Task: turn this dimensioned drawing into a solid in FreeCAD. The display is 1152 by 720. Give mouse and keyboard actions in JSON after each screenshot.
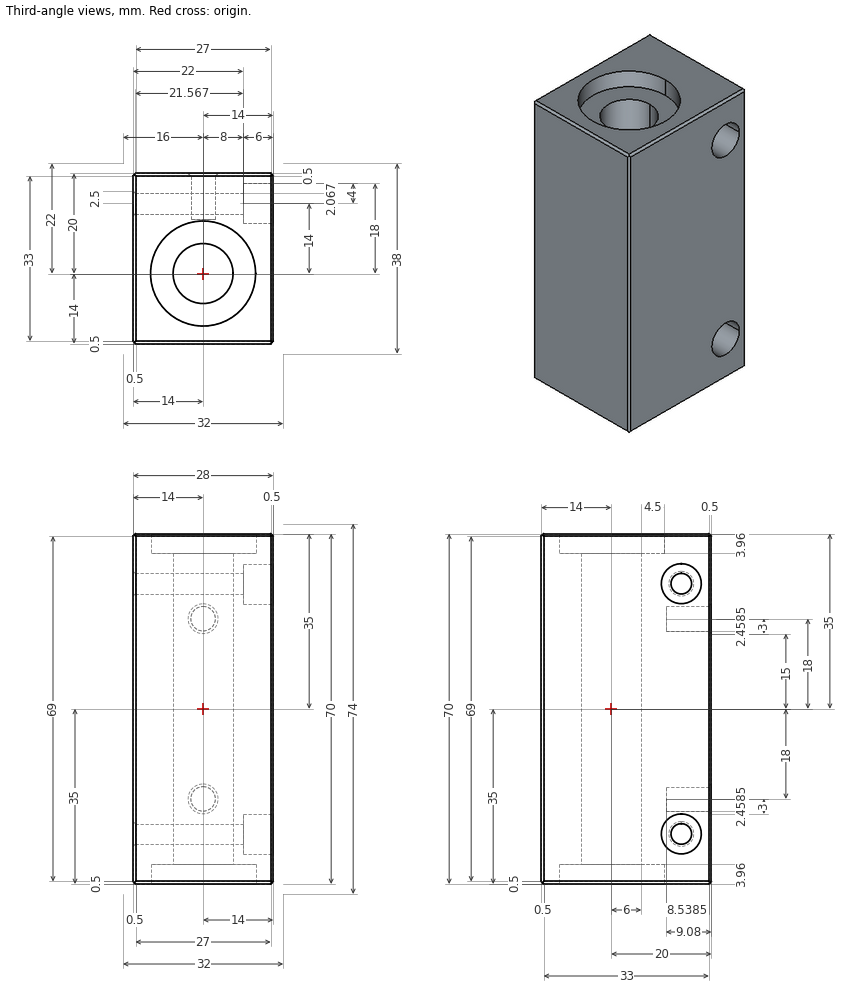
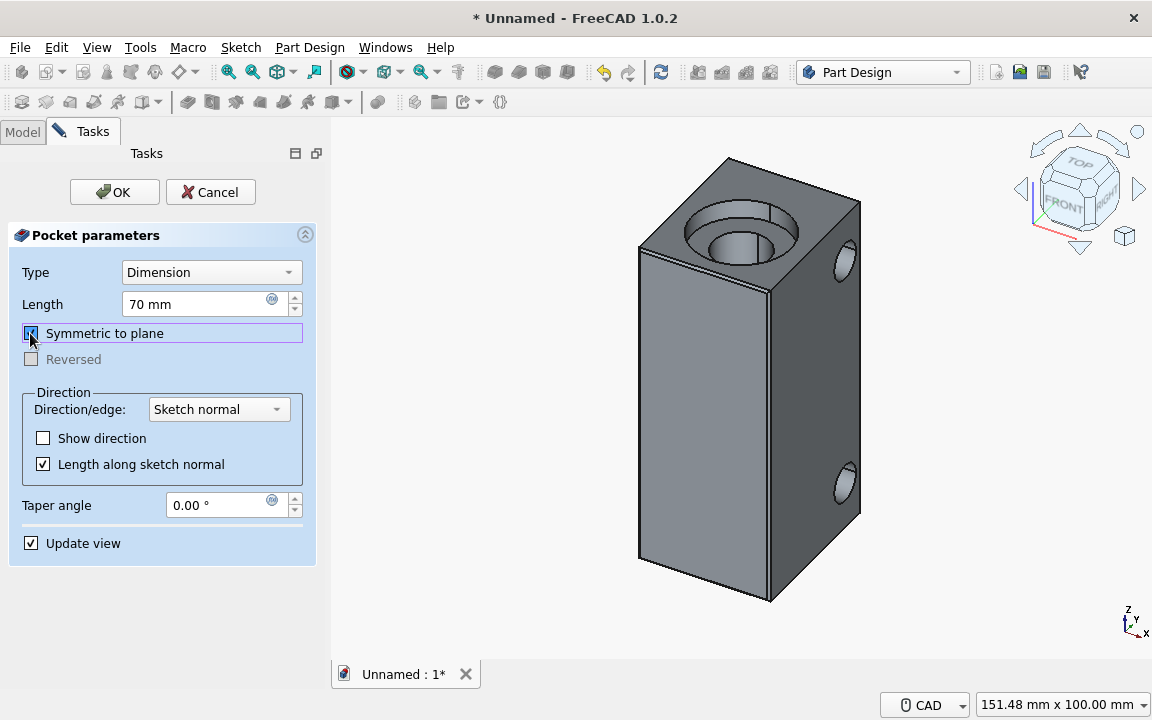
{"action": "left_click", "coordinate": [115, 192]}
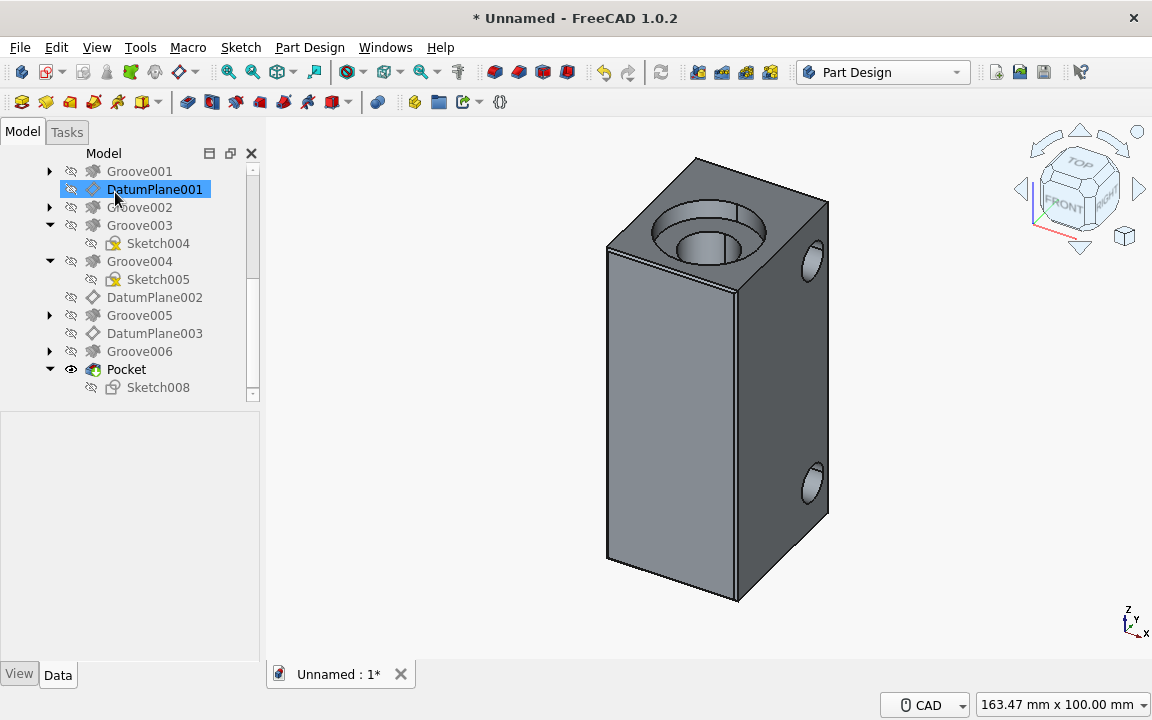
{"action": "left_click", "coordinate": [46, 72]}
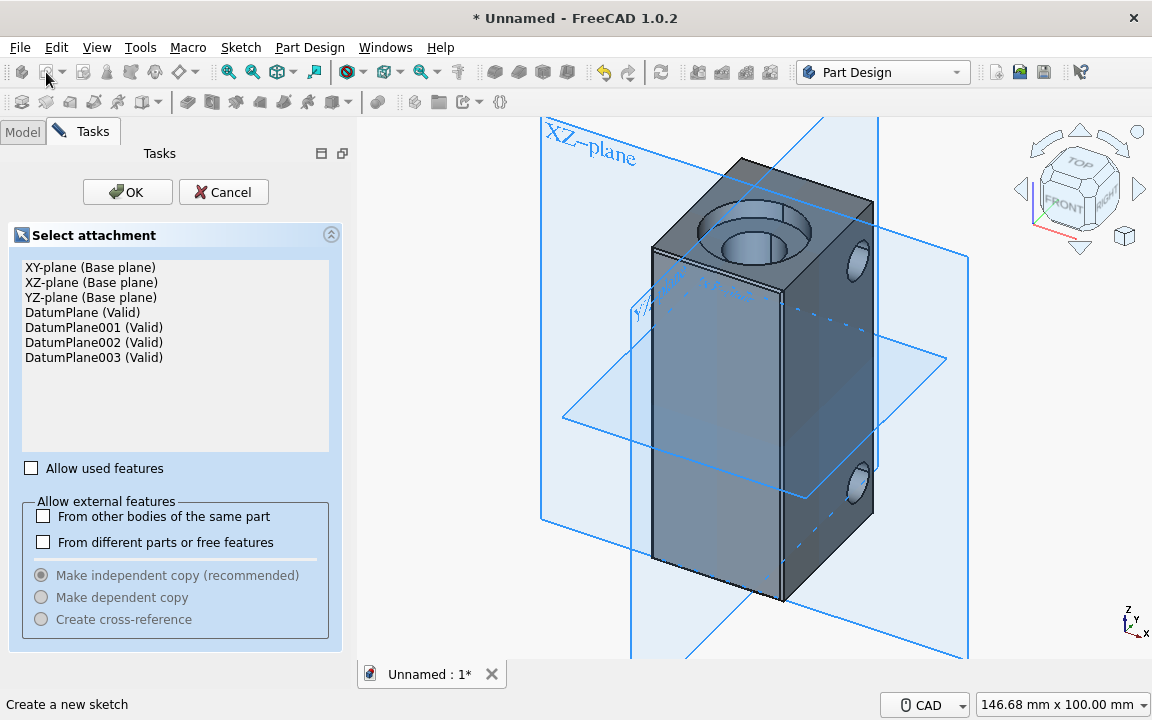
{"action": "left_click", "coordinate": [82, 282]}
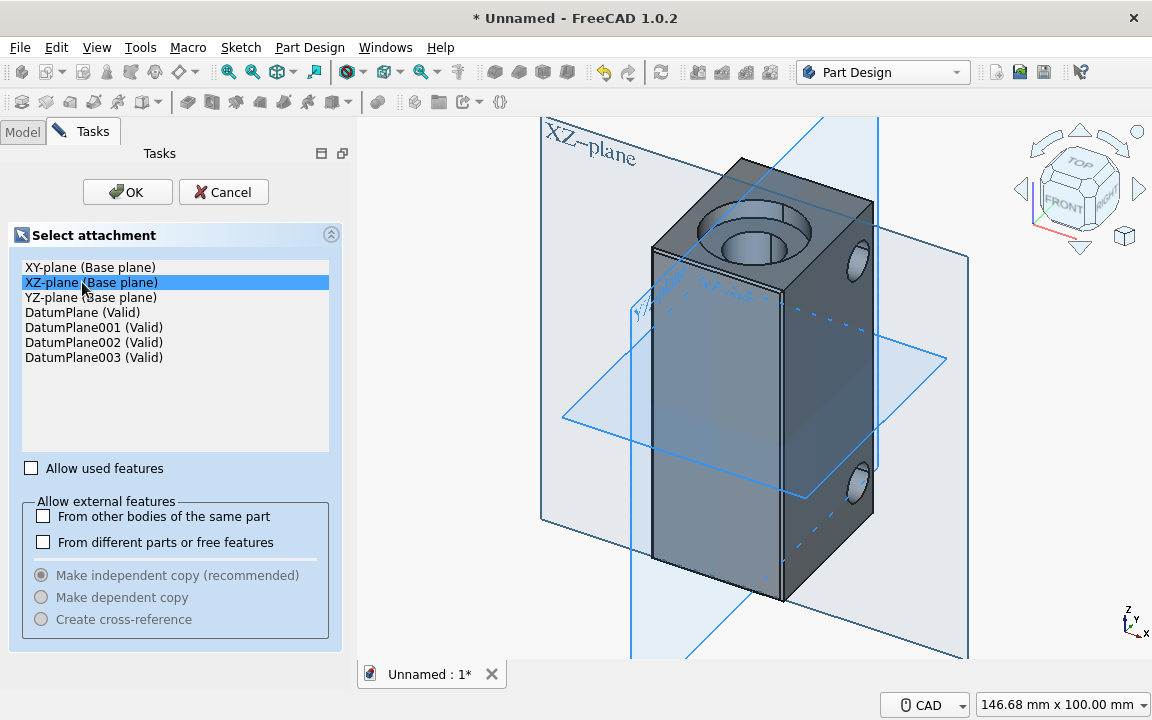
{"action": "left_click", "coordinate": [128, 192]}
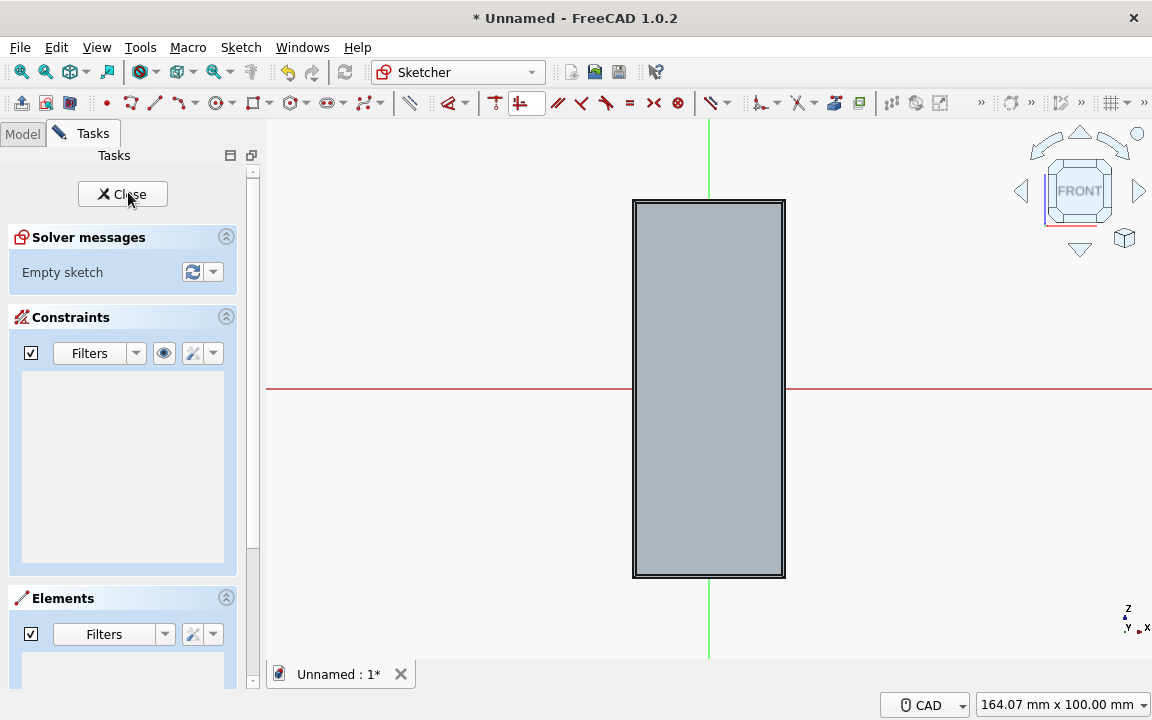
{"action": "left_click", "coordinate": [70, 104]}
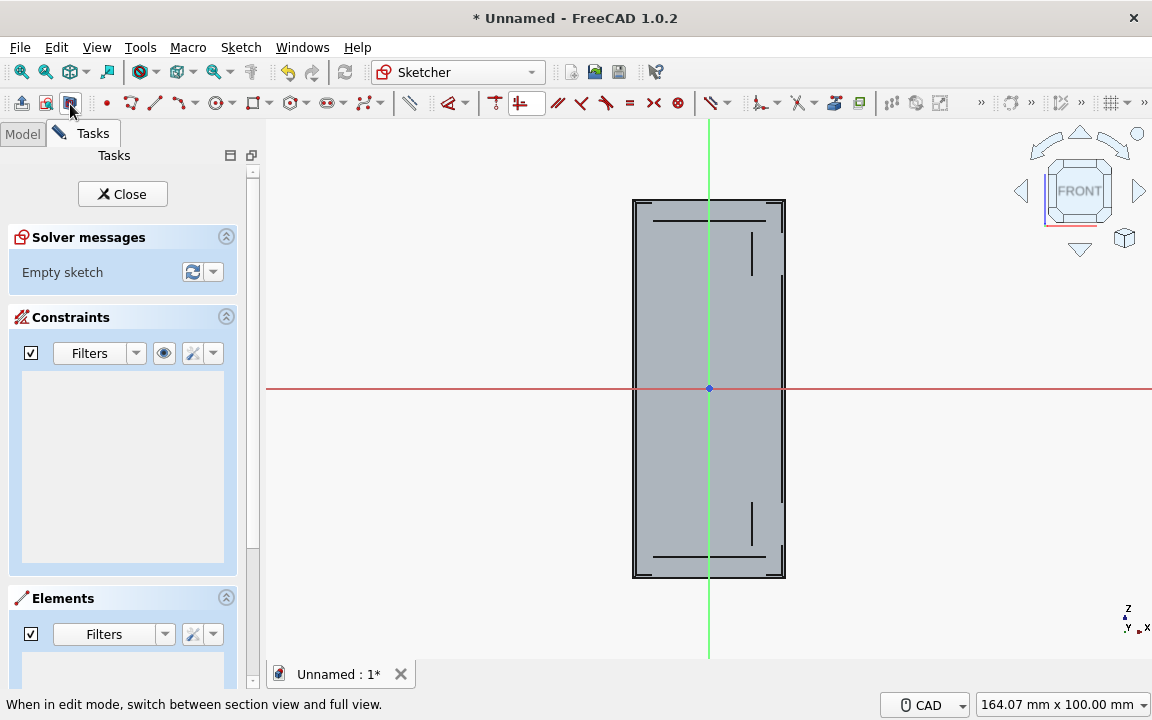
{"action": "left_click", "coordinate": [272, 104]}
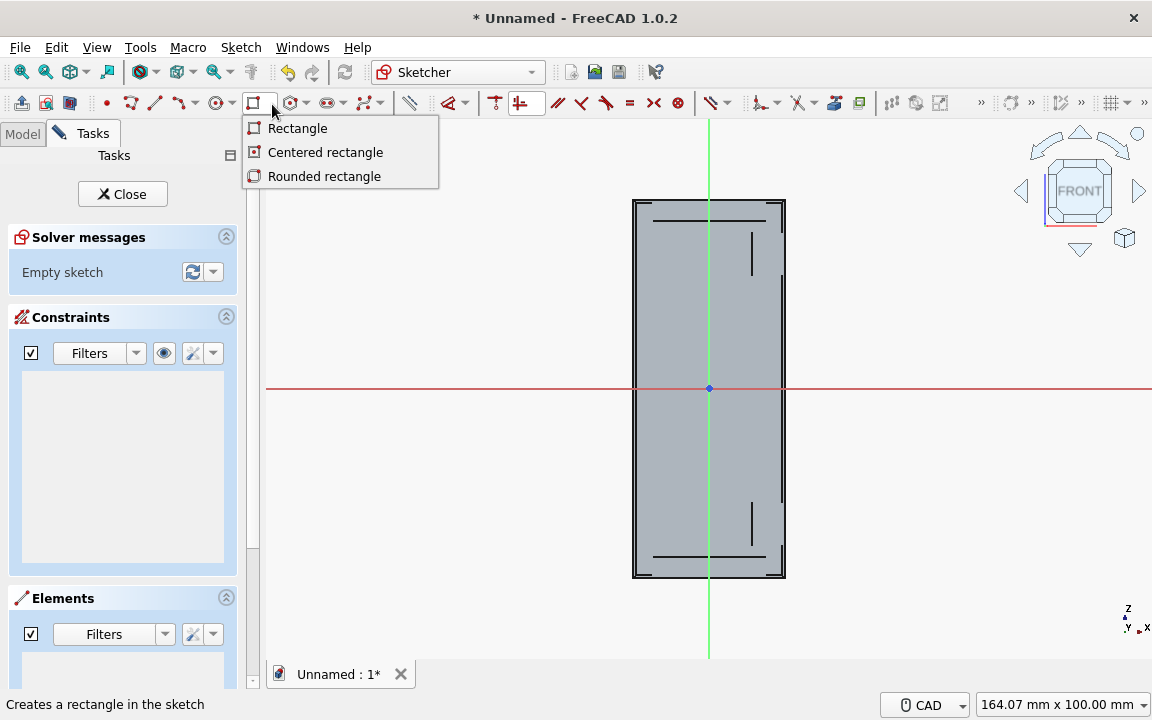
{"action": "left_click", "coordinate": [340, 152]}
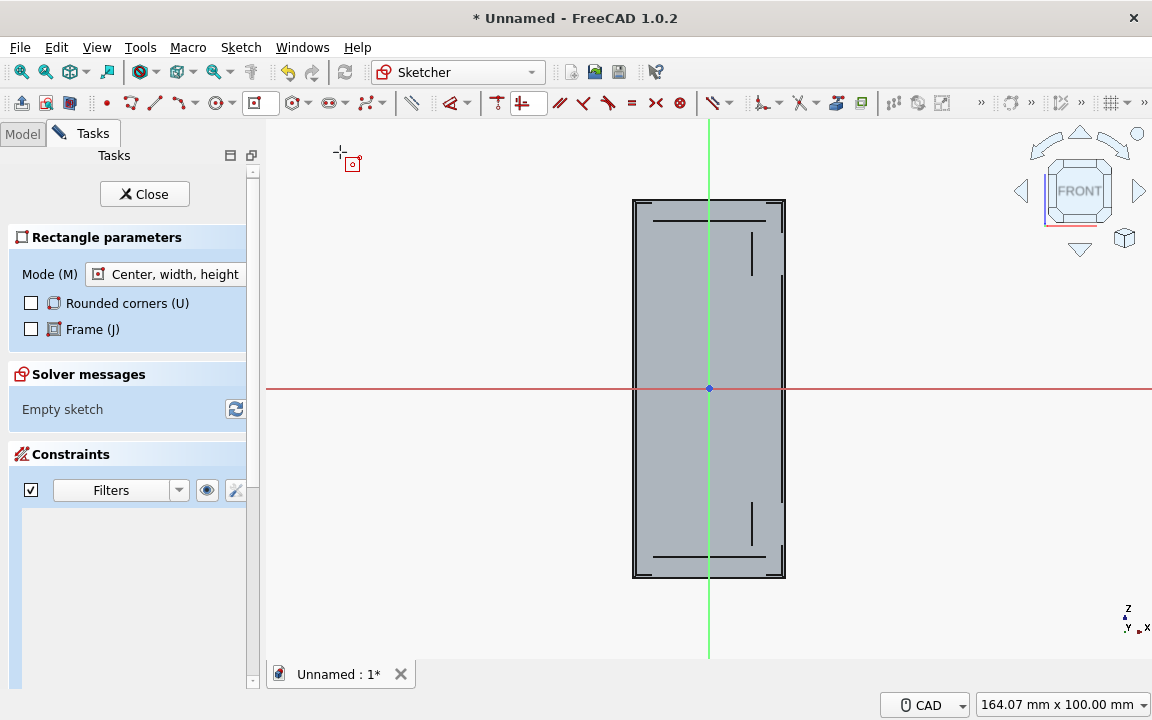
{"action": "left_click", "coordinate": [709, 389]}
{"action": "mouse_move", "coordinate": [795, 189]}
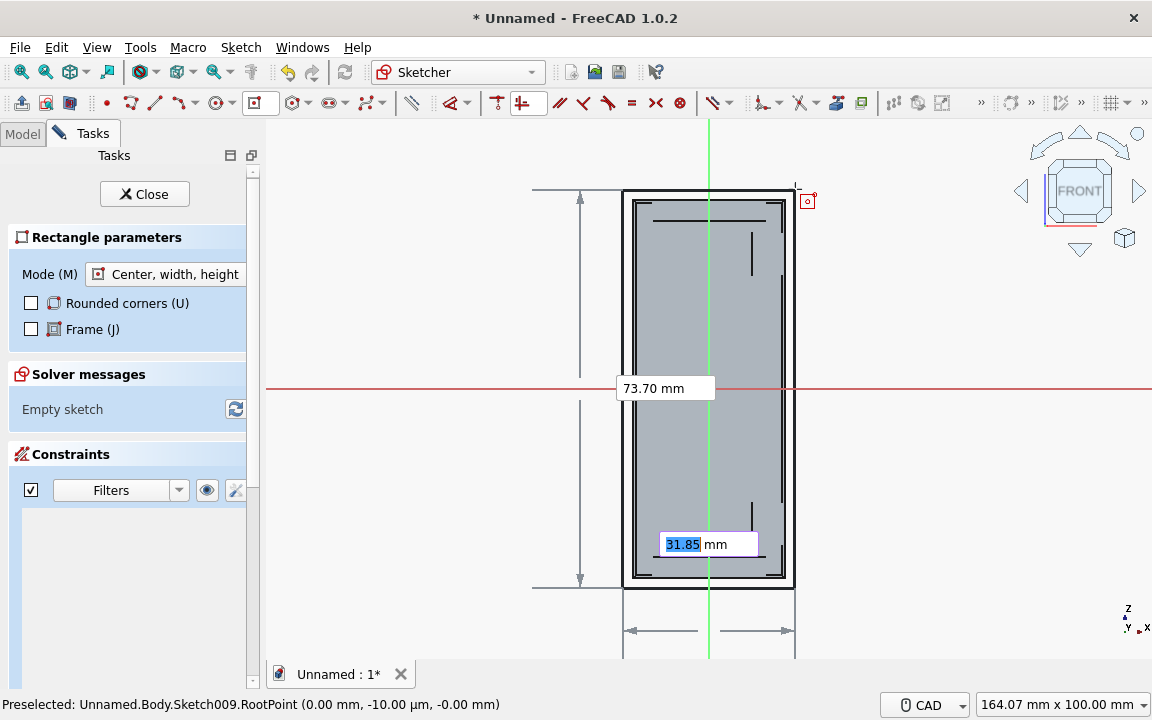
{"action": "type", "text": "32"}
{"action": "key", "text": "Tab"}
{"action": "type", "text": "74"}
{"action": "key", "text": "Return"}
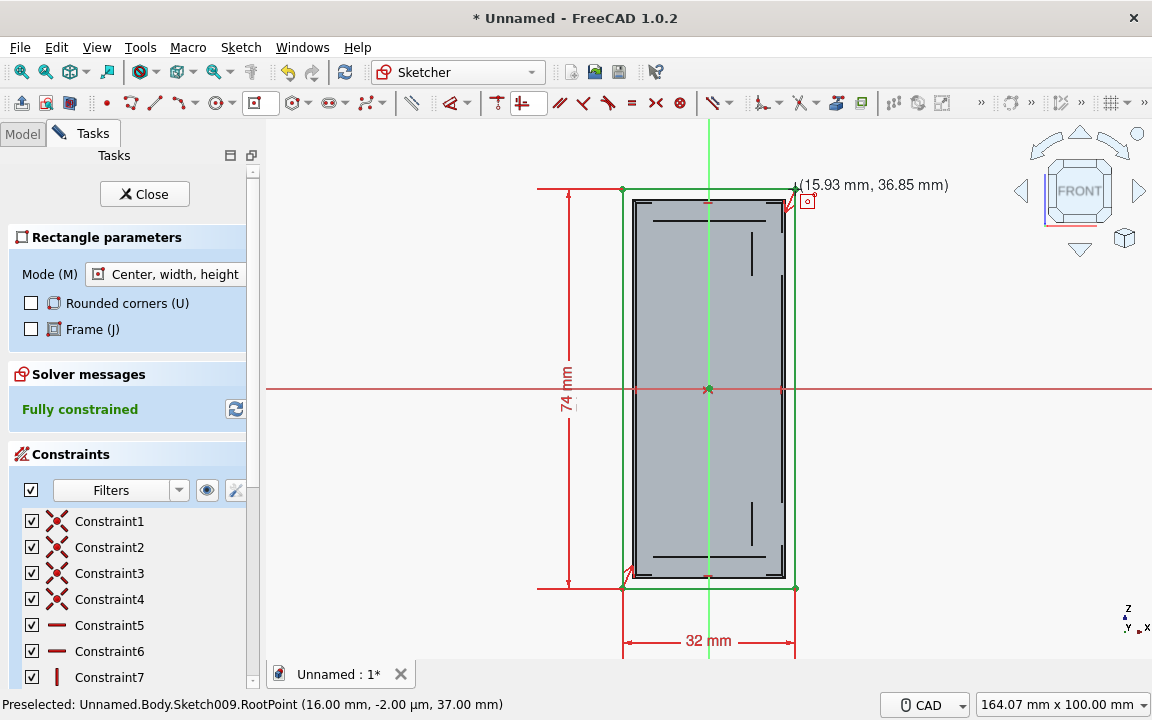
{"action": "left_click", "coordinate": [132, 104]}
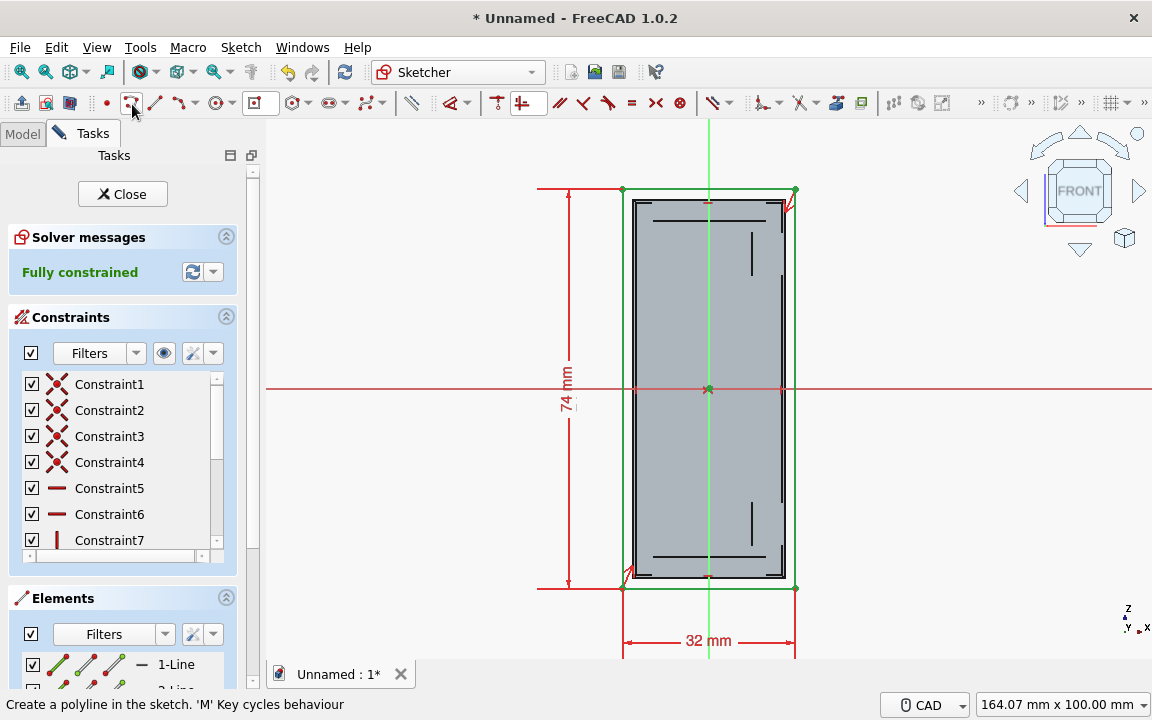
{"action": "scroll", "coordinate": [633, 203], "scroll_direction": "up", "scroll_amount": 2}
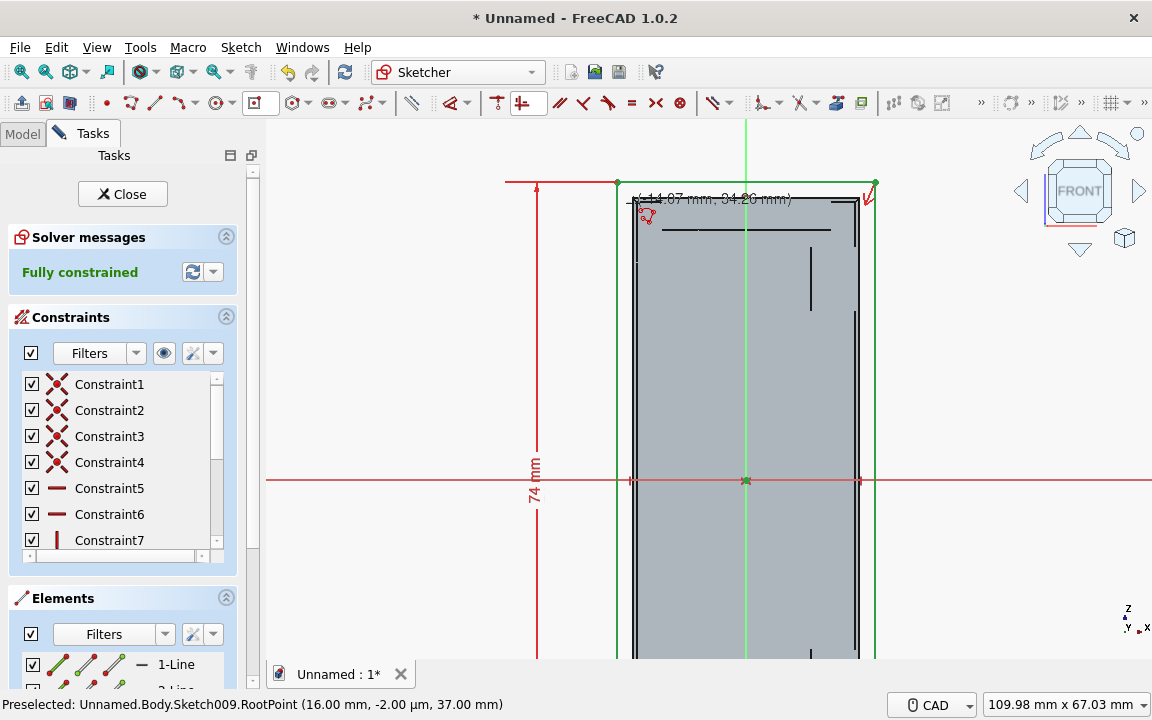
{"action": "left_click", "coordinate": [633, 202]}